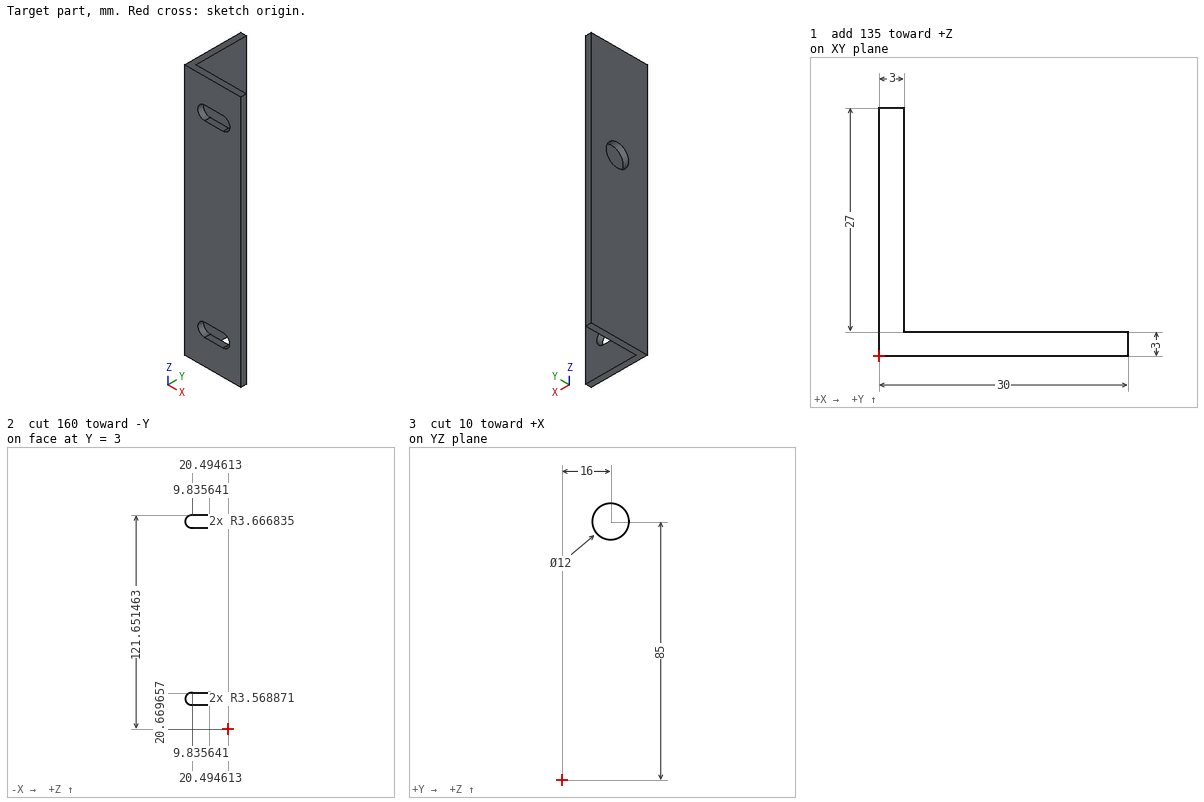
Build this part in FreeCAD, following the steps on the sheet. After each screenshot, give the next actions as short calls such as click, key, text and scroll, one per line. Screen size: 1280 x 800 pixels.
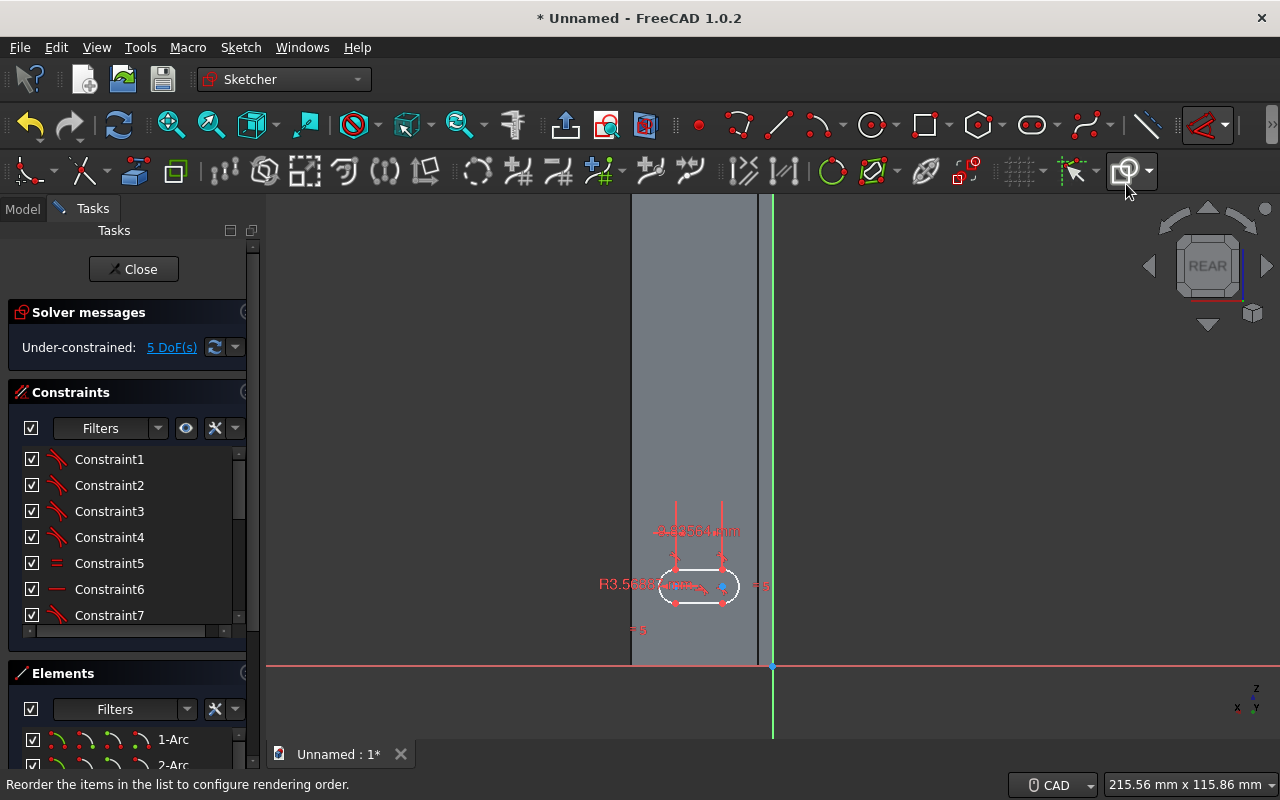
scroll(691, 571, down, 3)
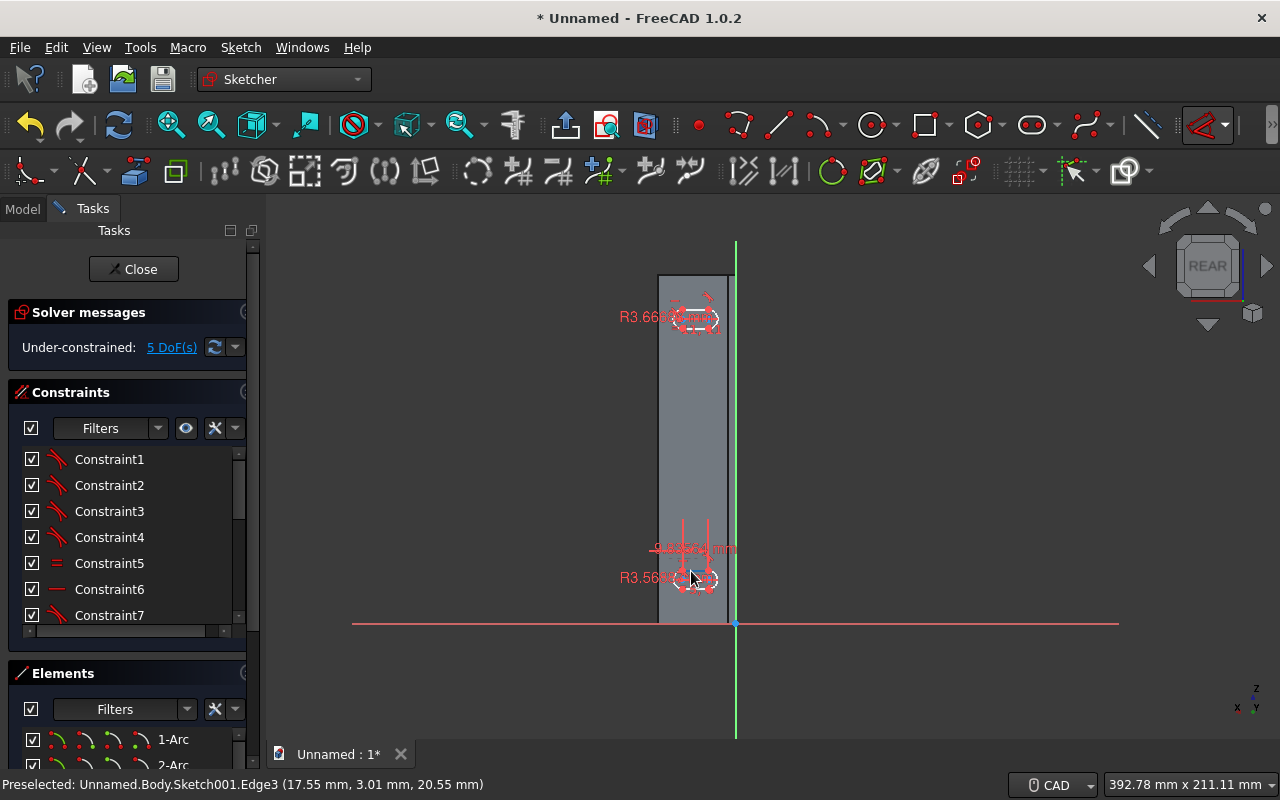
scroll(691, 310, up, 3)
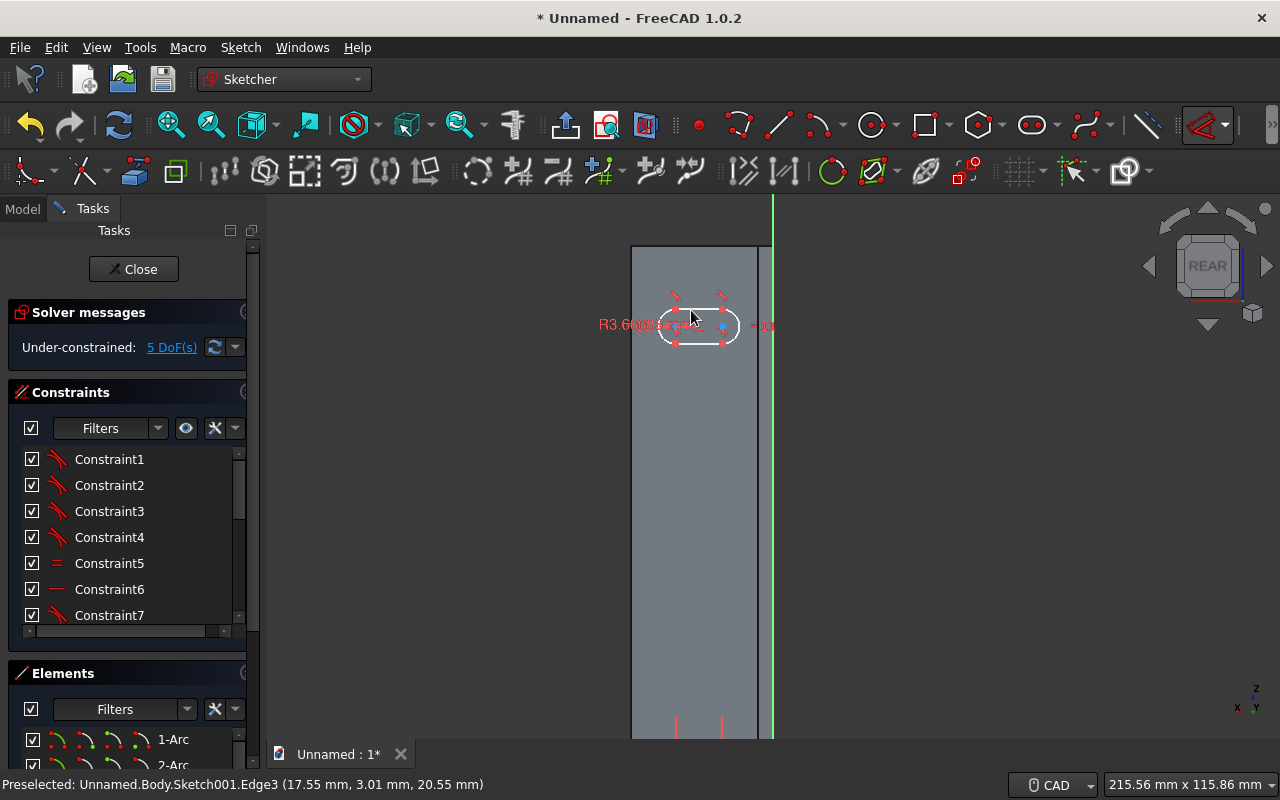
click(690, 309)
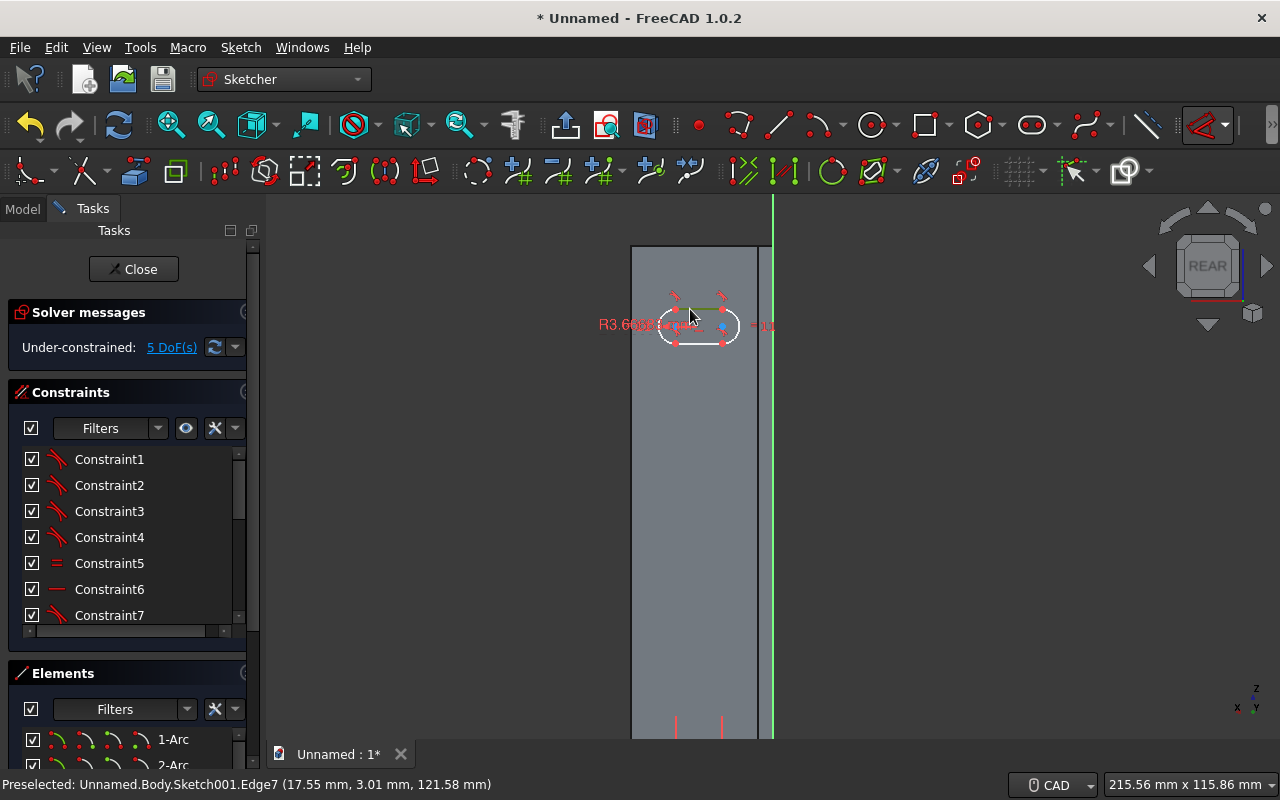
key(l)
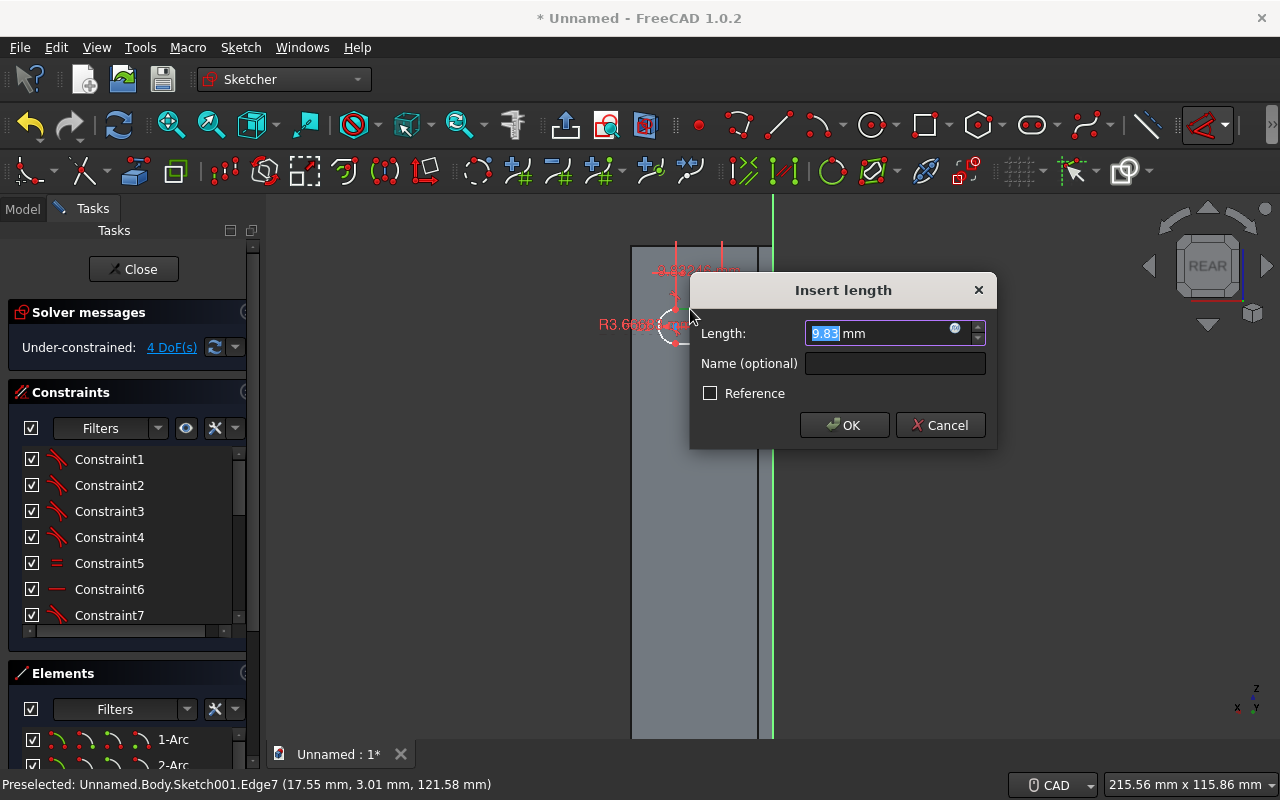
text(9.835641)
key(Return)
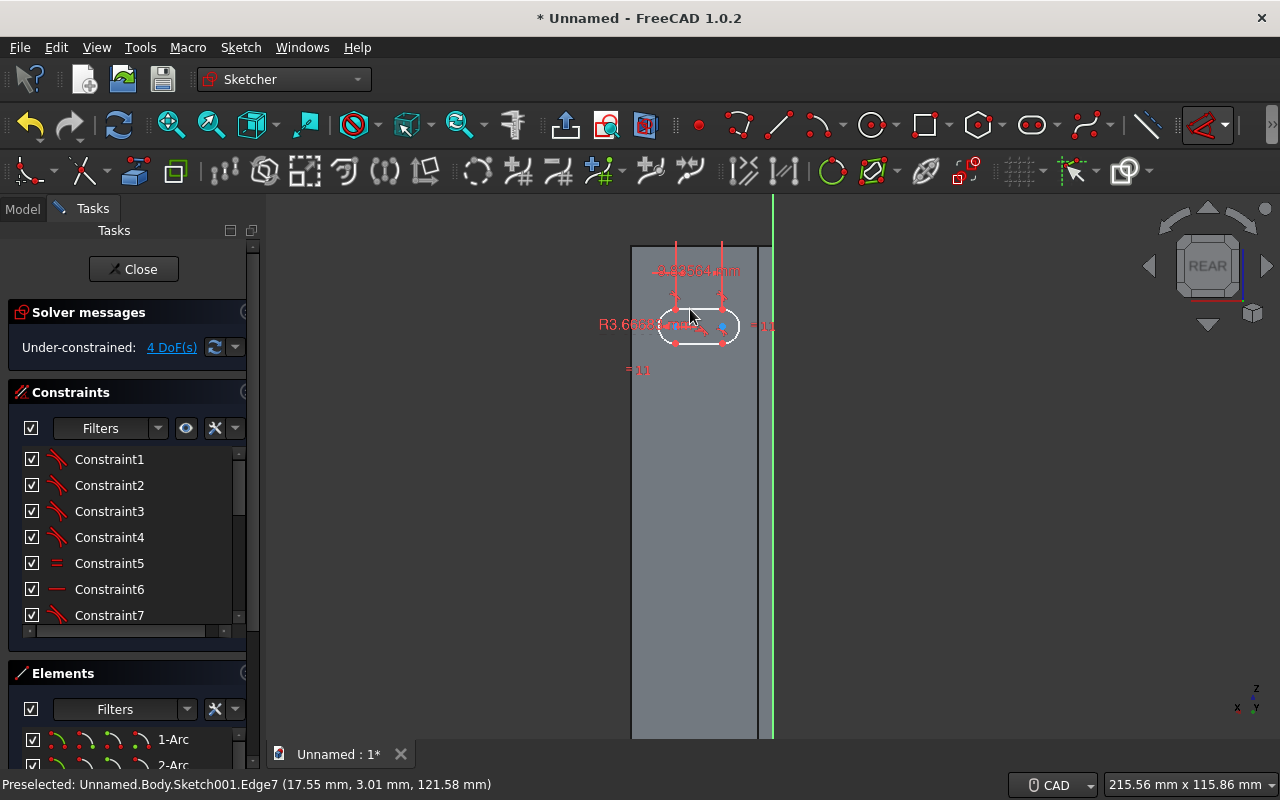
scroll(691, 310, down, 3)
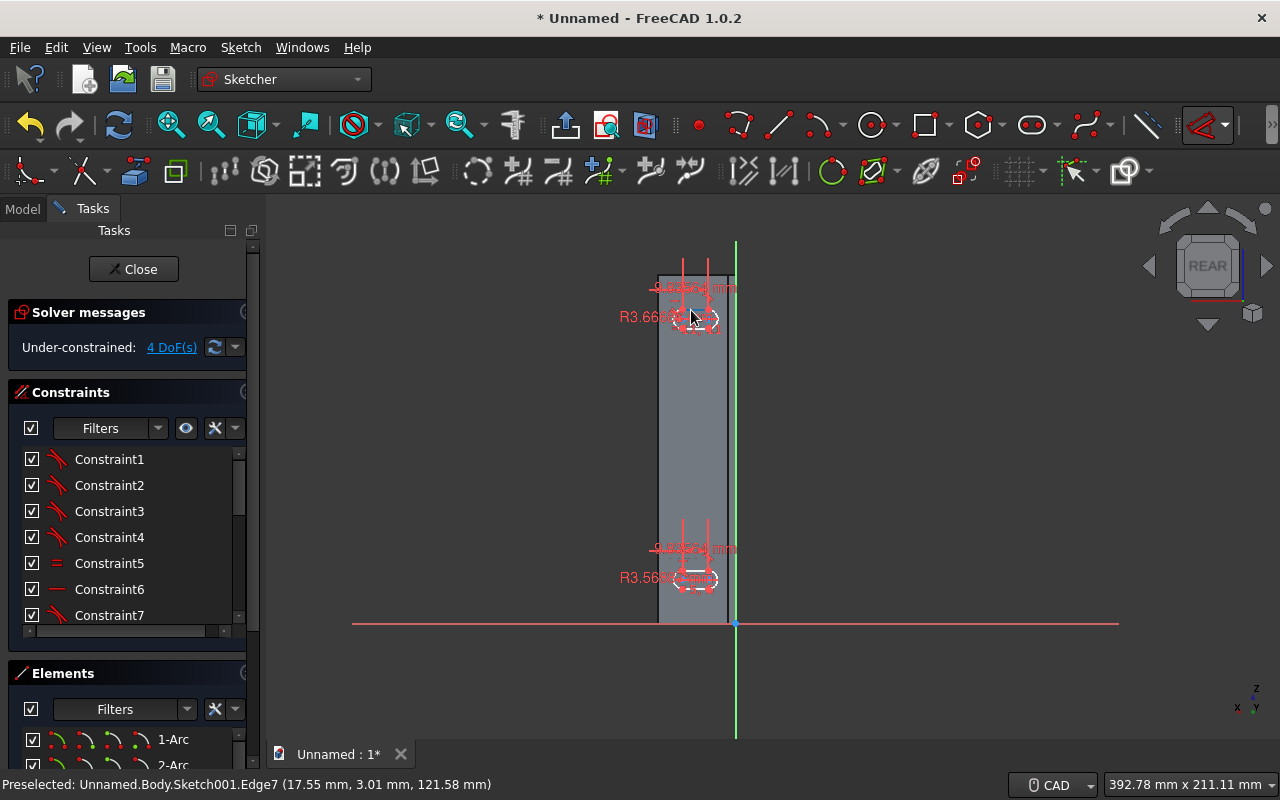
scroll(683, 571, up, 2)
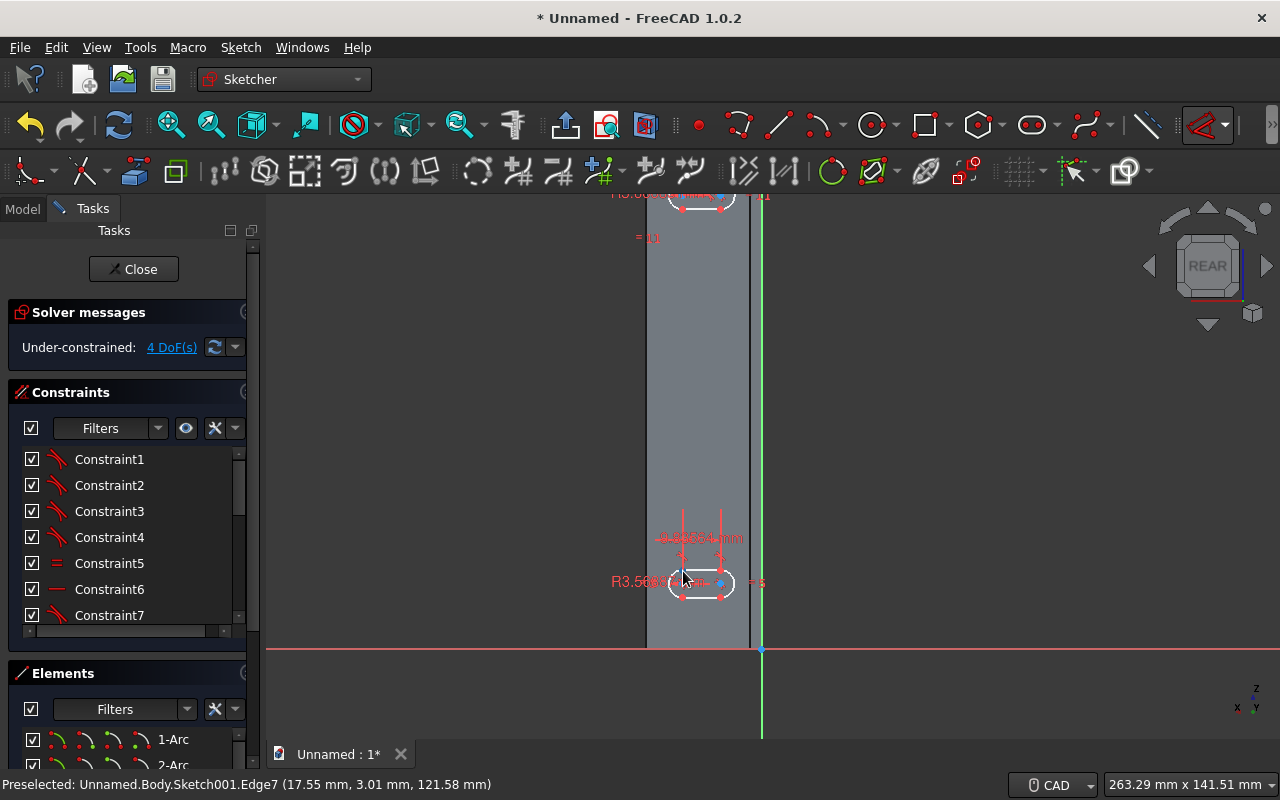
click(683, 570)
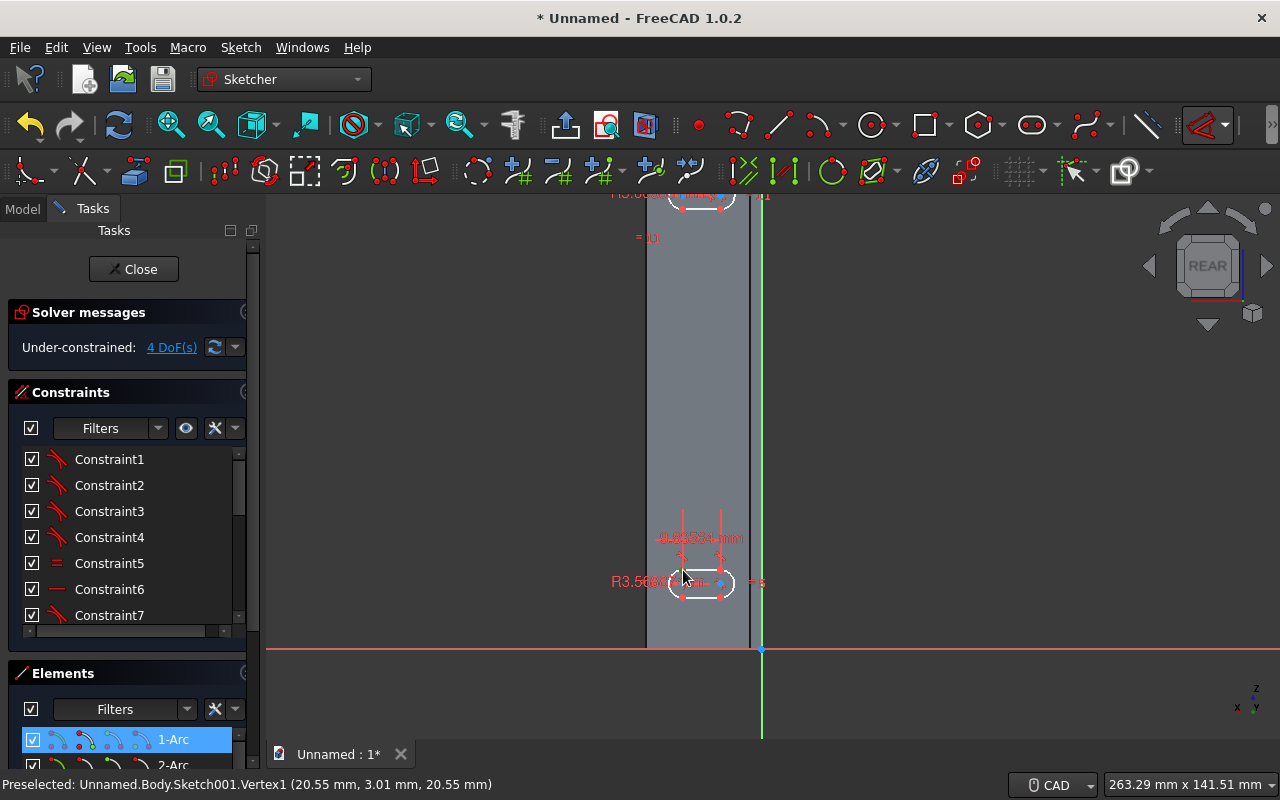
key(l)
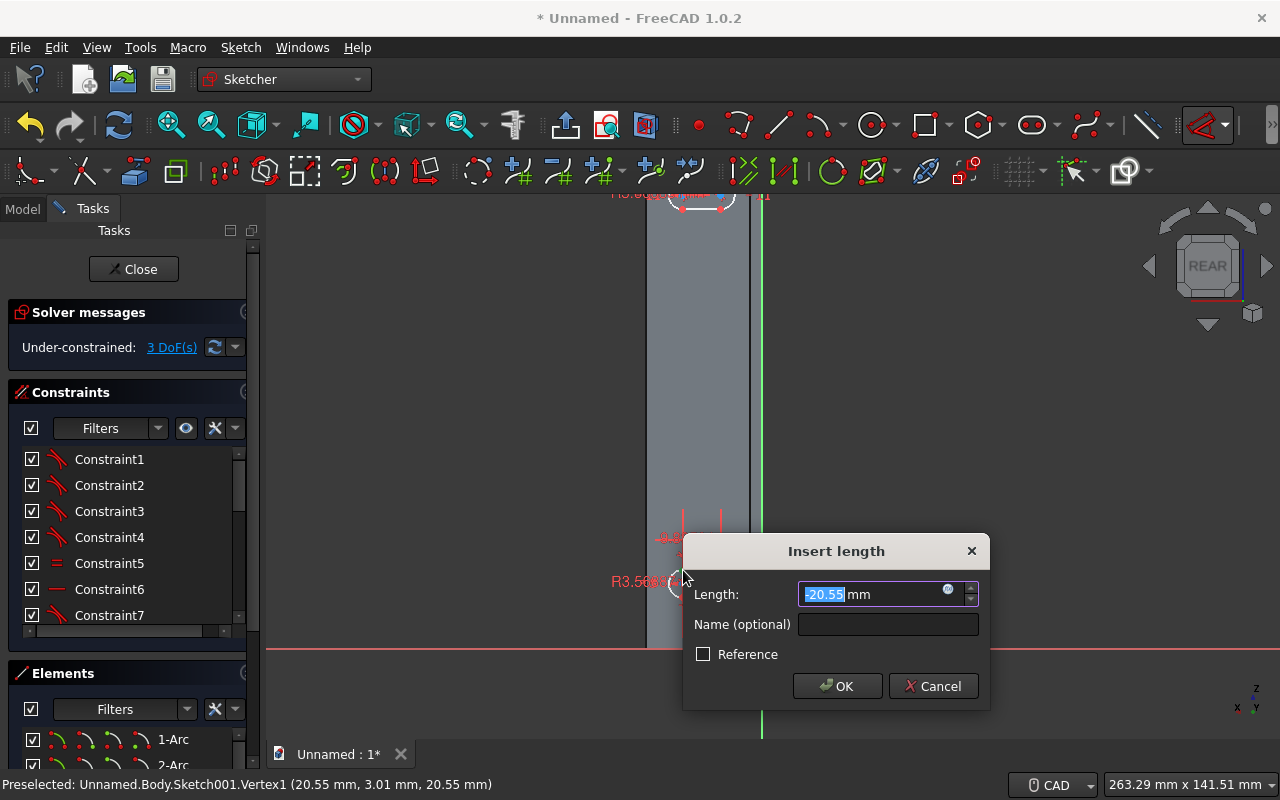
text(-20.494613)
key(Return)